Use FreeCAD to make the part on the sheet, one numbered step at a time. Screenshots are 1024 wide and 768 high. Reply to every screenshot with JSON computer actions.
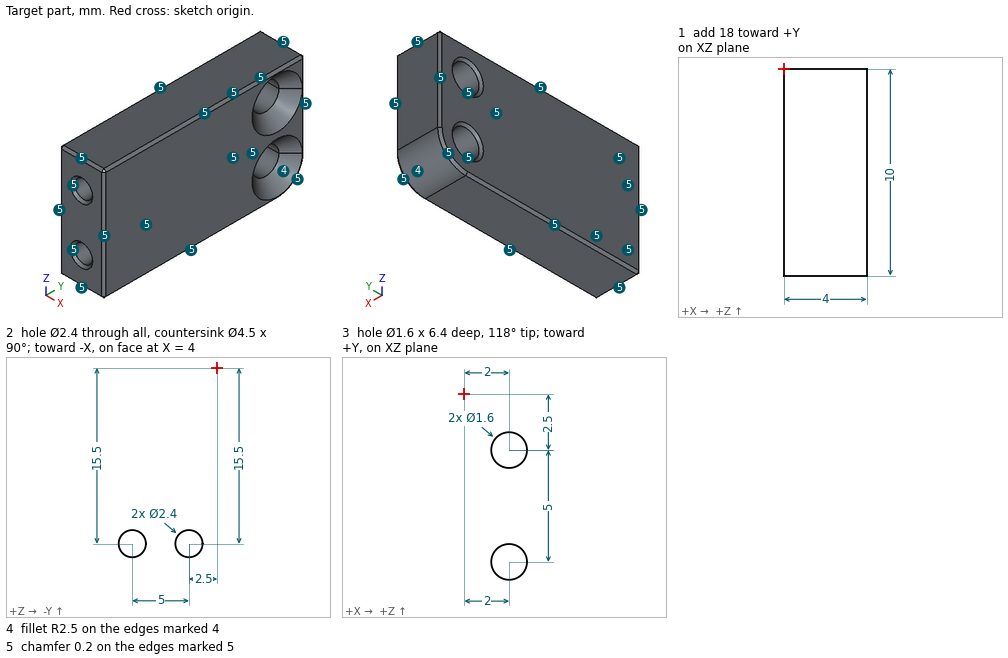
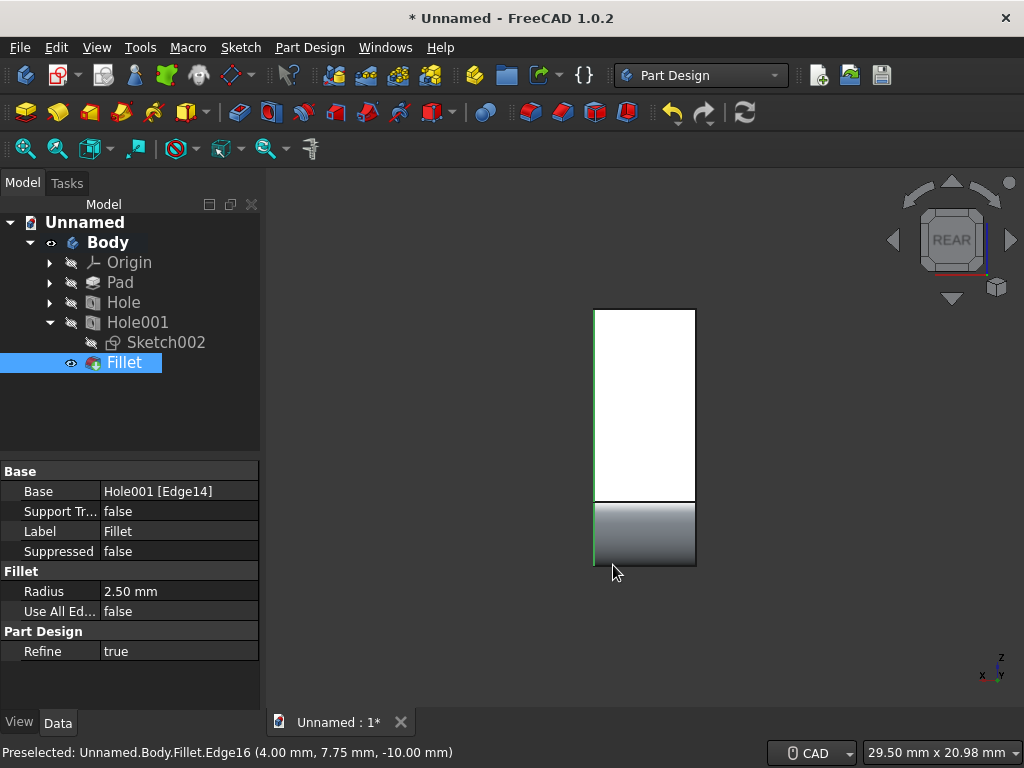
{"action": "key", "text": "6"}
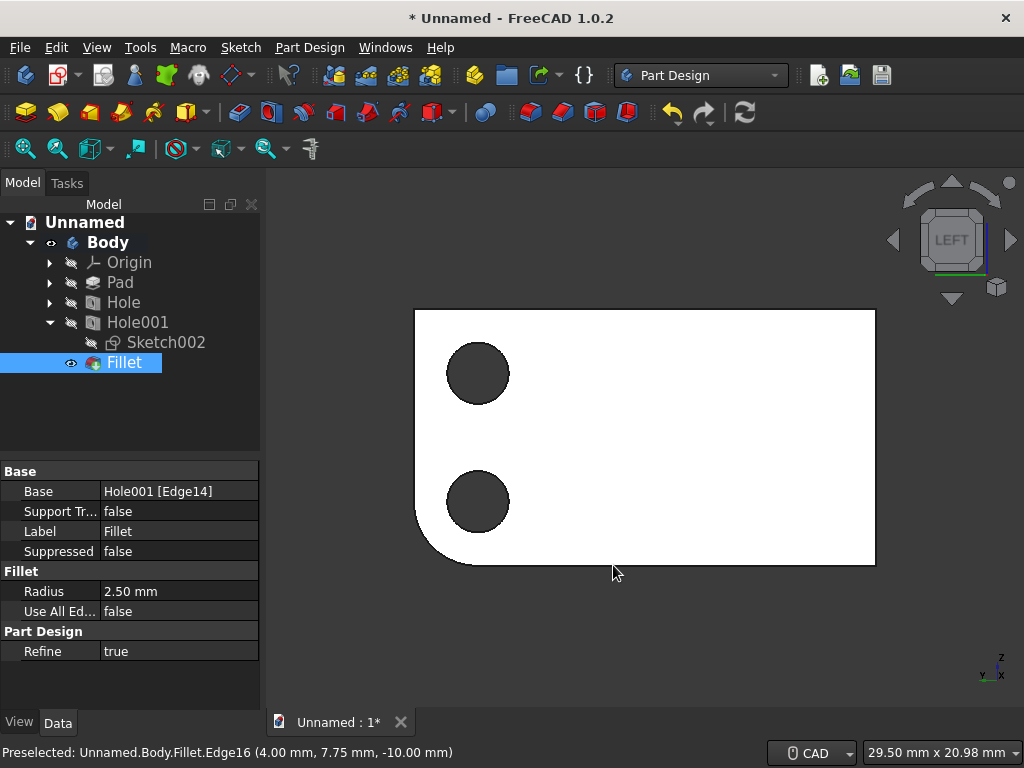
{"action": "left_click", "coordinate": [711, 436], "text": "ctrl"}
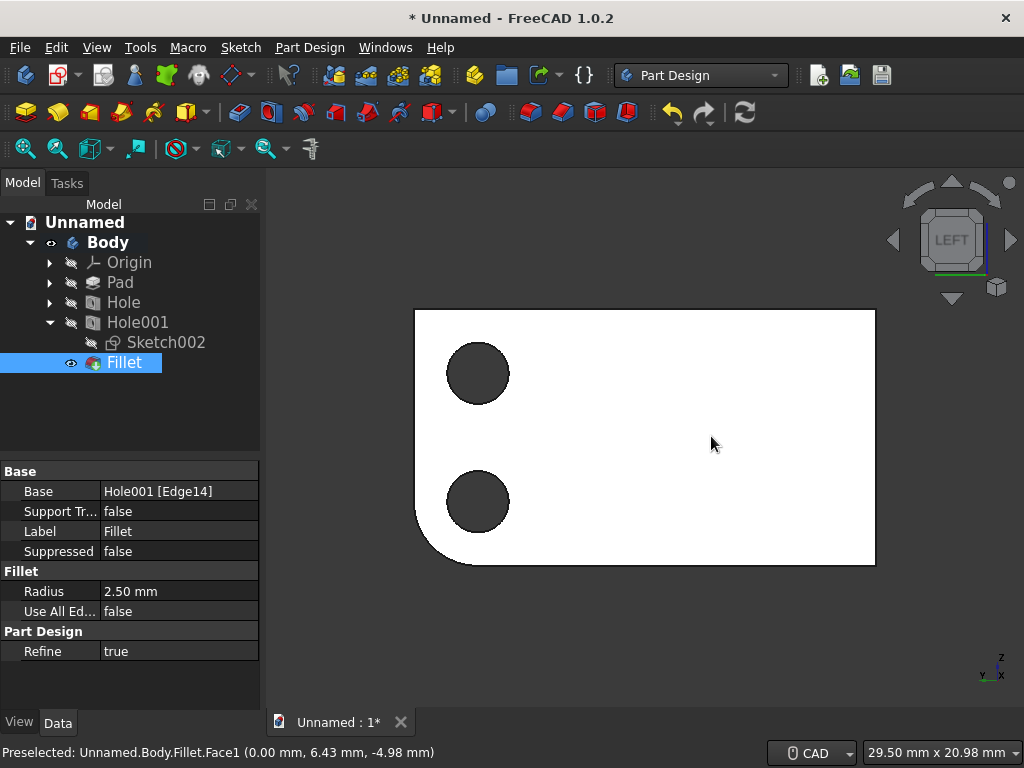
{"action": "left_click", "coordinate": [564, 112]}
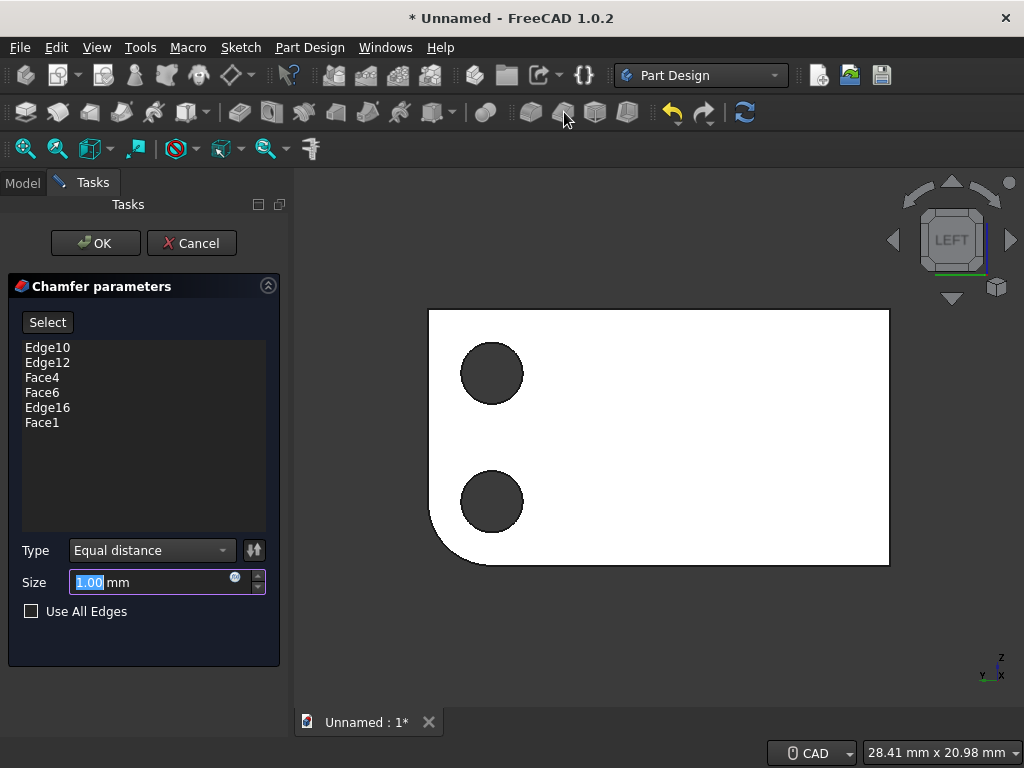
{"action": "type", "text": "0.2"}
{"action": "key", "text": "Tab"}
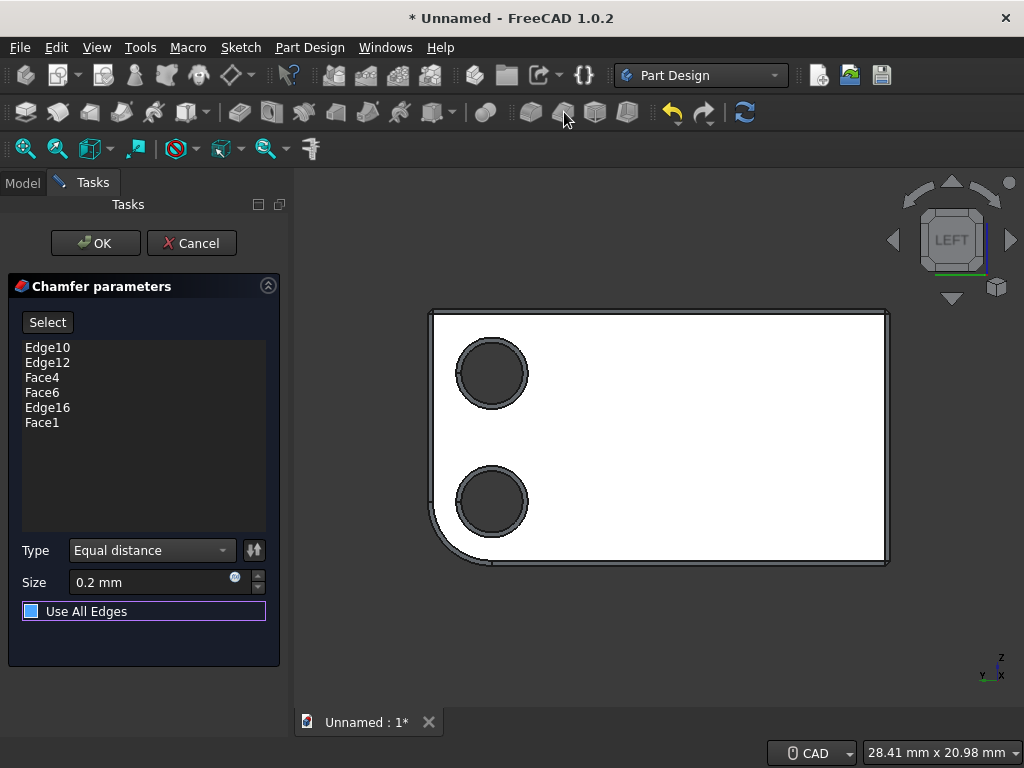
{"action": "left_click", "coordinate": [96, 243]}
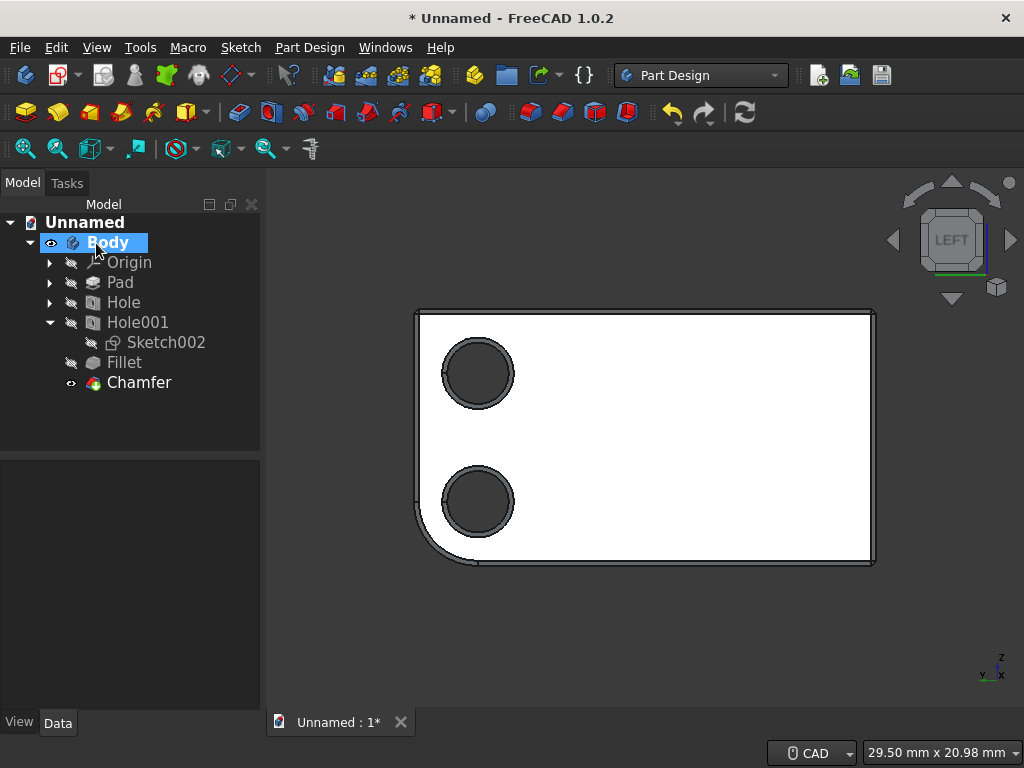
{"action": "key", "text": "0"}